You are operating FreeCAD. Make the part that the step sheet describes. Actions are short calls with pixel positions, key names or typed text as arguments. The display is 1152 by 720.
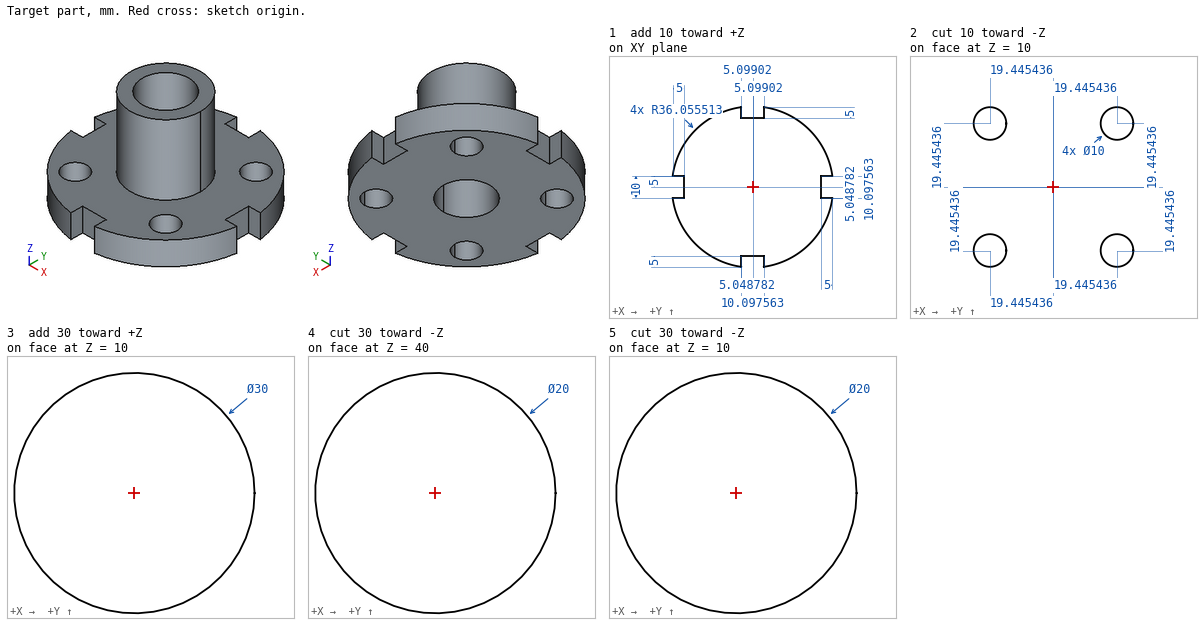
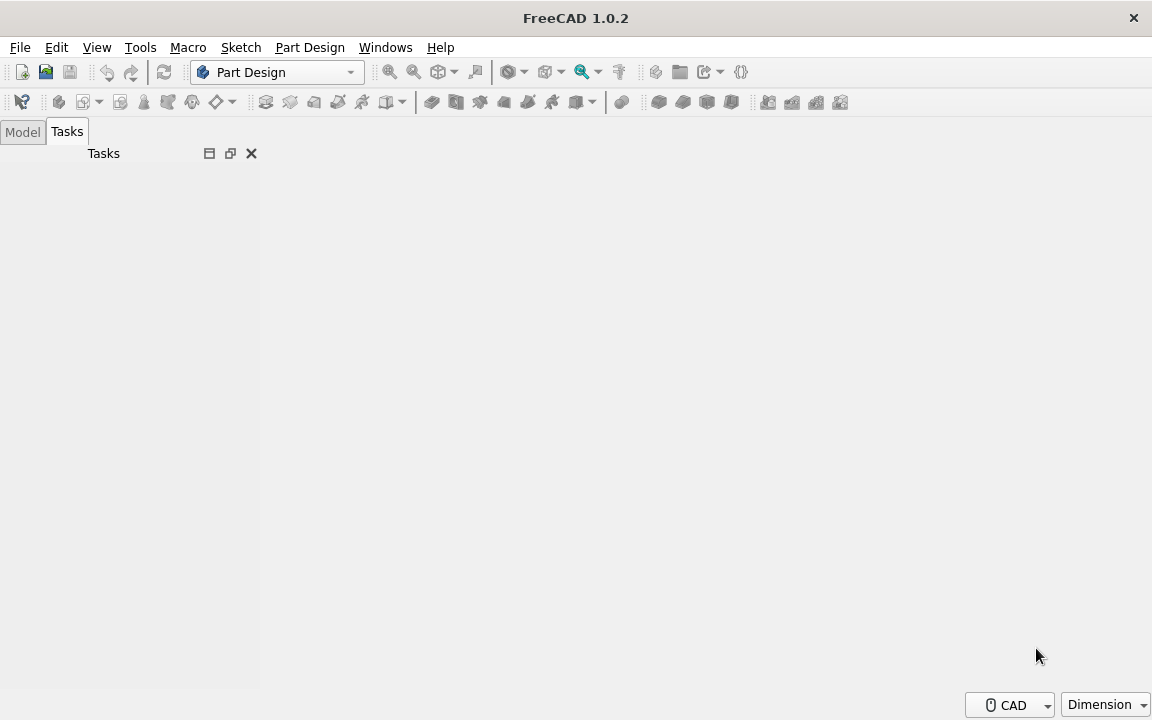
click(22, 72)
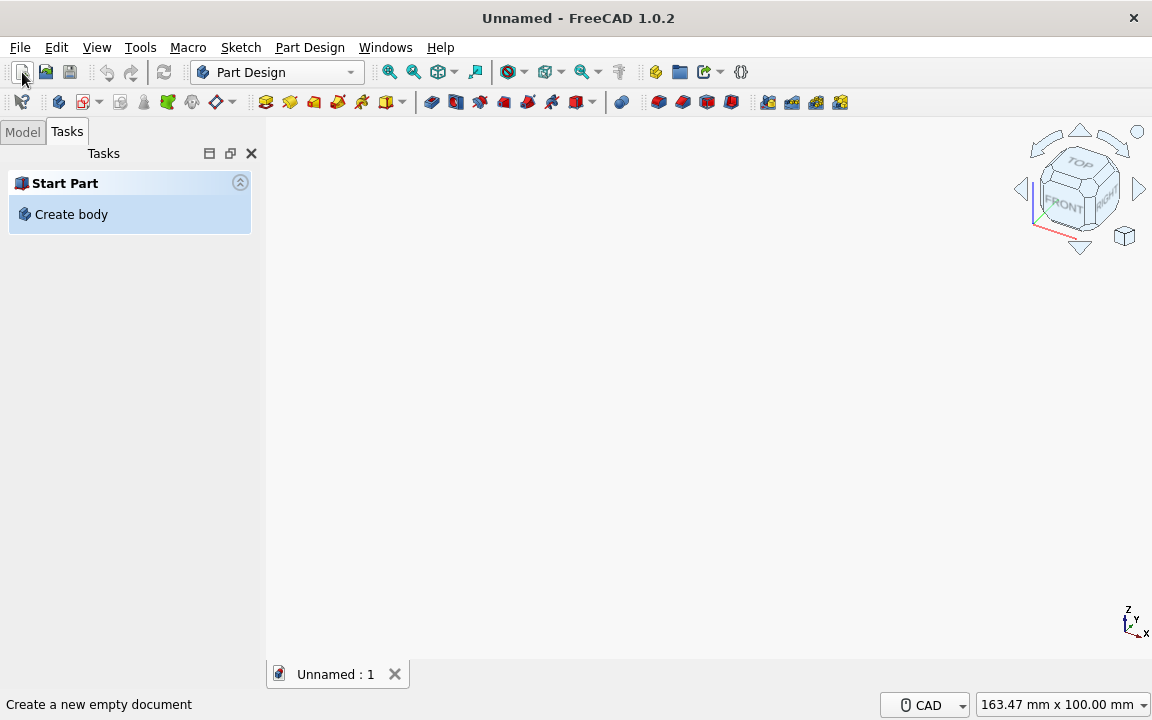
click(84, 102)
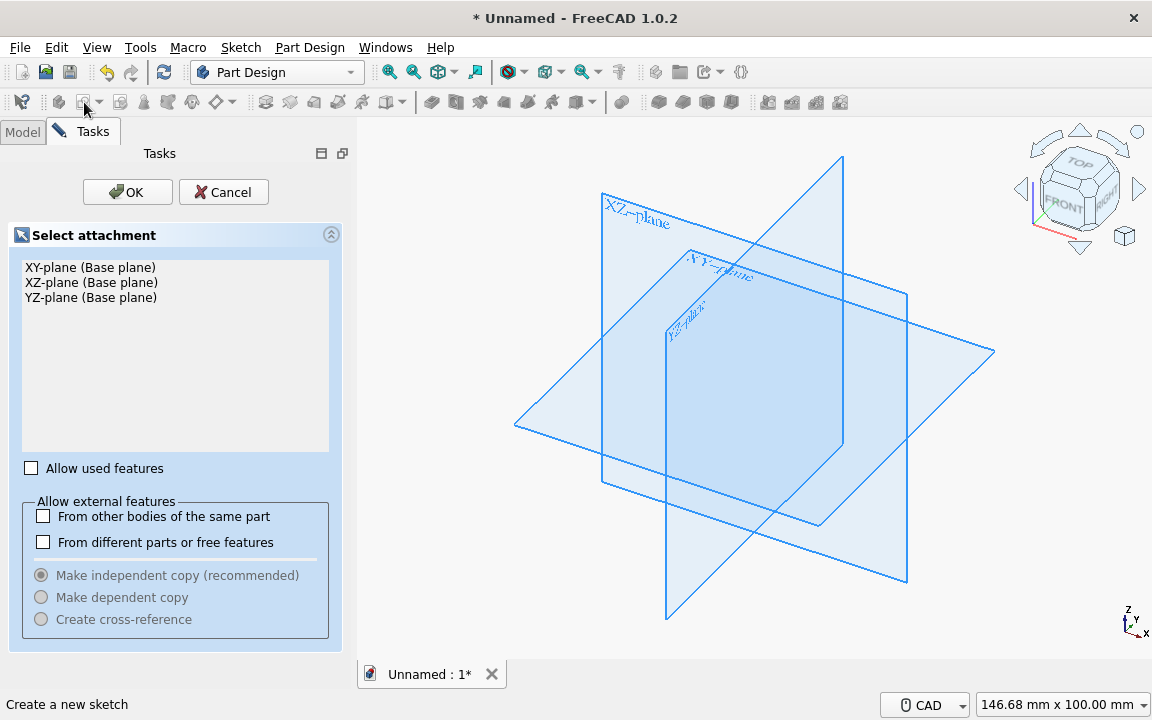
click(82, 268)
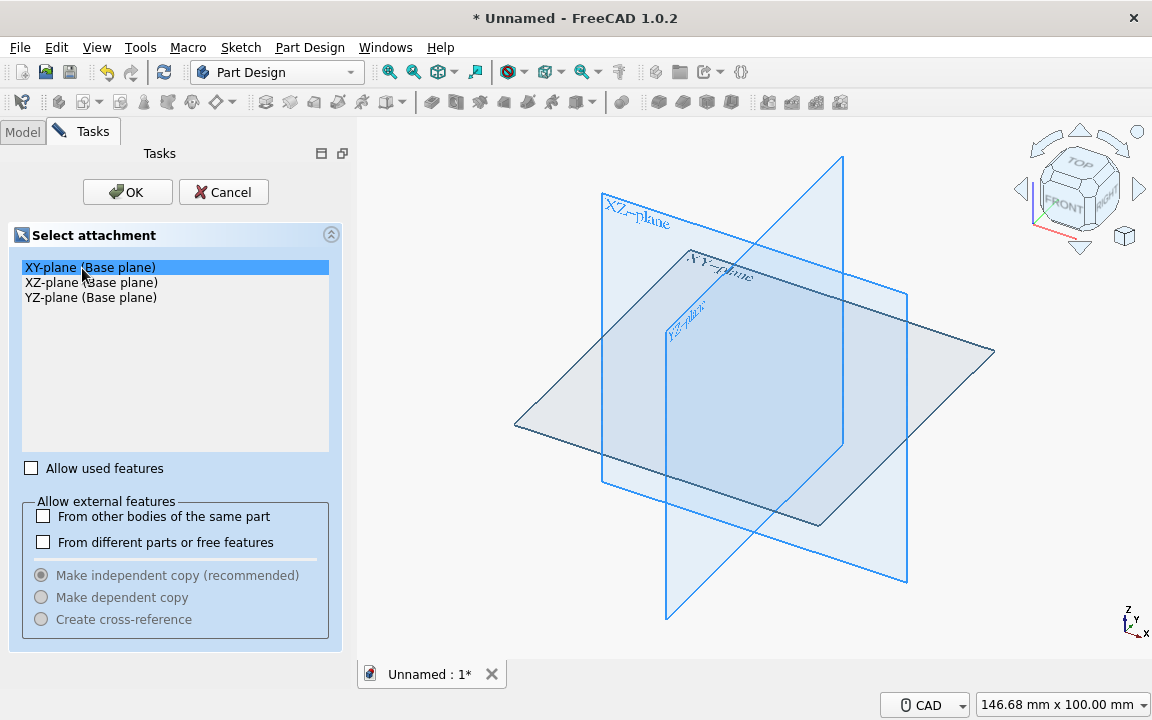
click(128, 192)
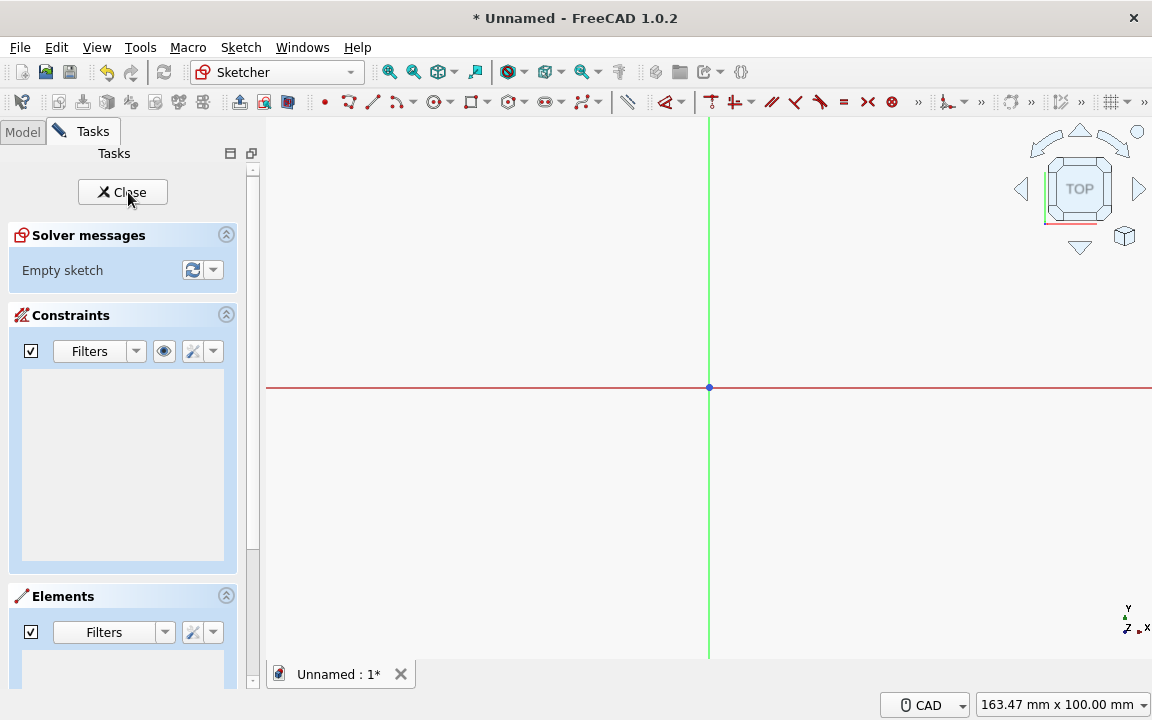
key(g)
key(m)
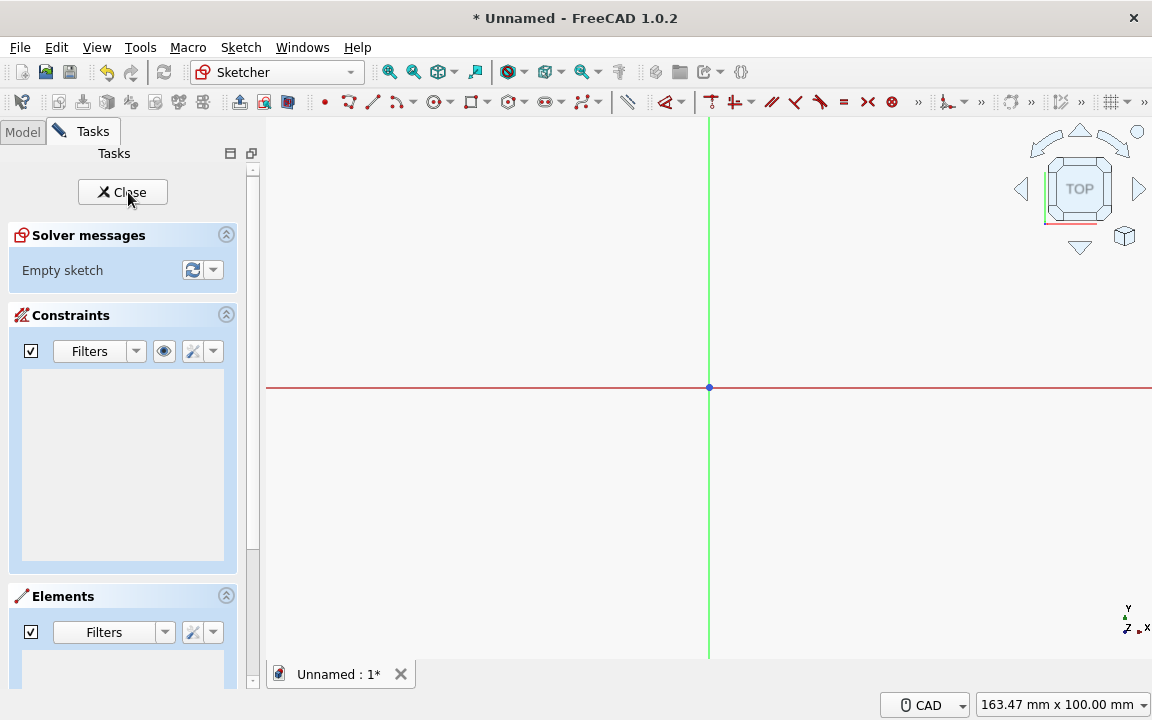
click(737, 195)
click(737, 222)
click(681, 222)
click(681, 195)
right_click(681, 195)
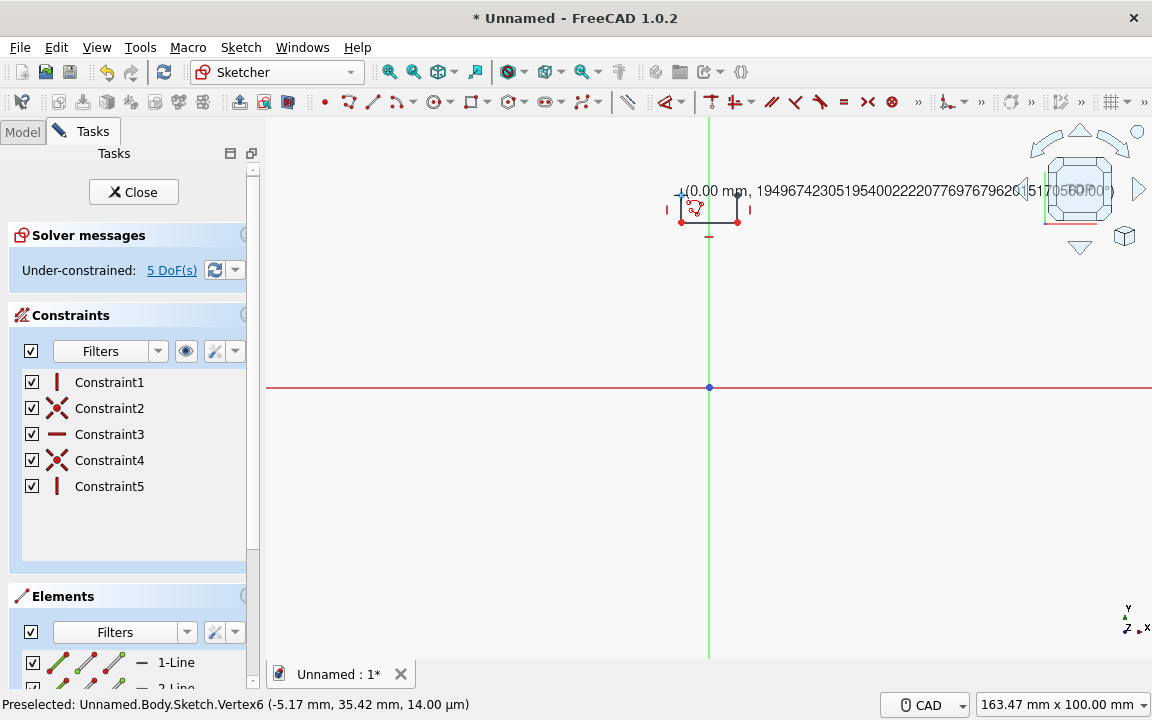
click(515, 361)
click(543, 361)
click(543, 415)
click(515, 415)
right_click(515, 415)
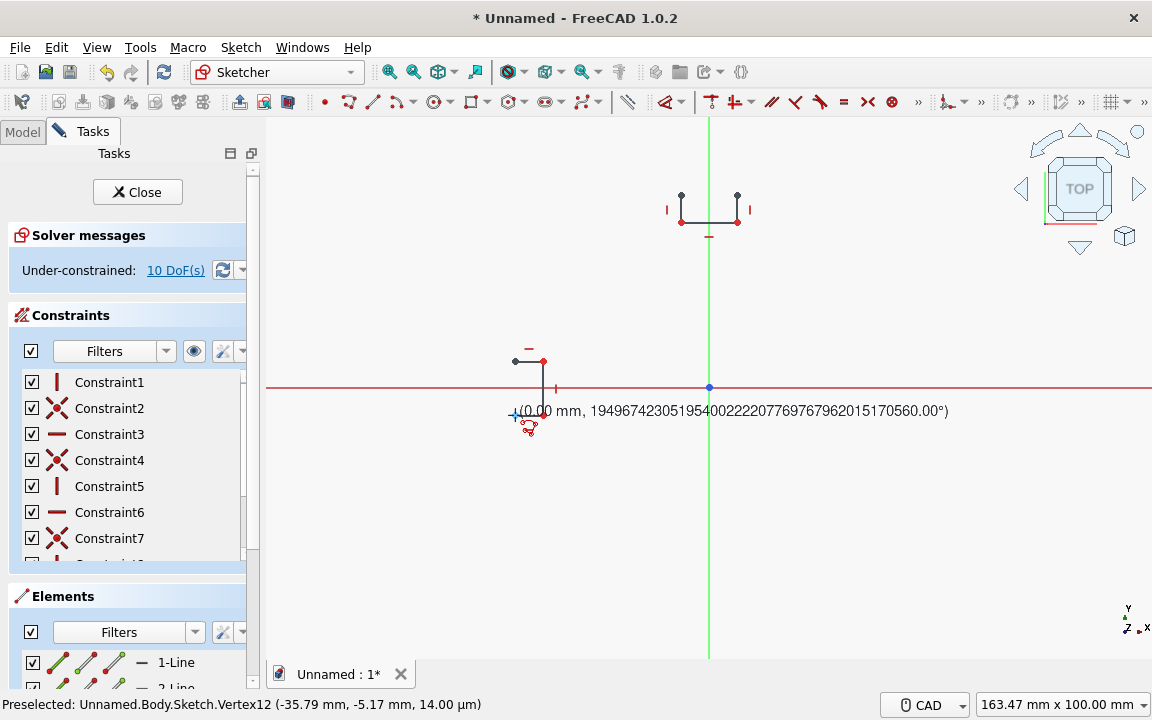
click(682, 581)
click(682, 554)
click(736, 554)
click(736, 581)
right_click(736, 581)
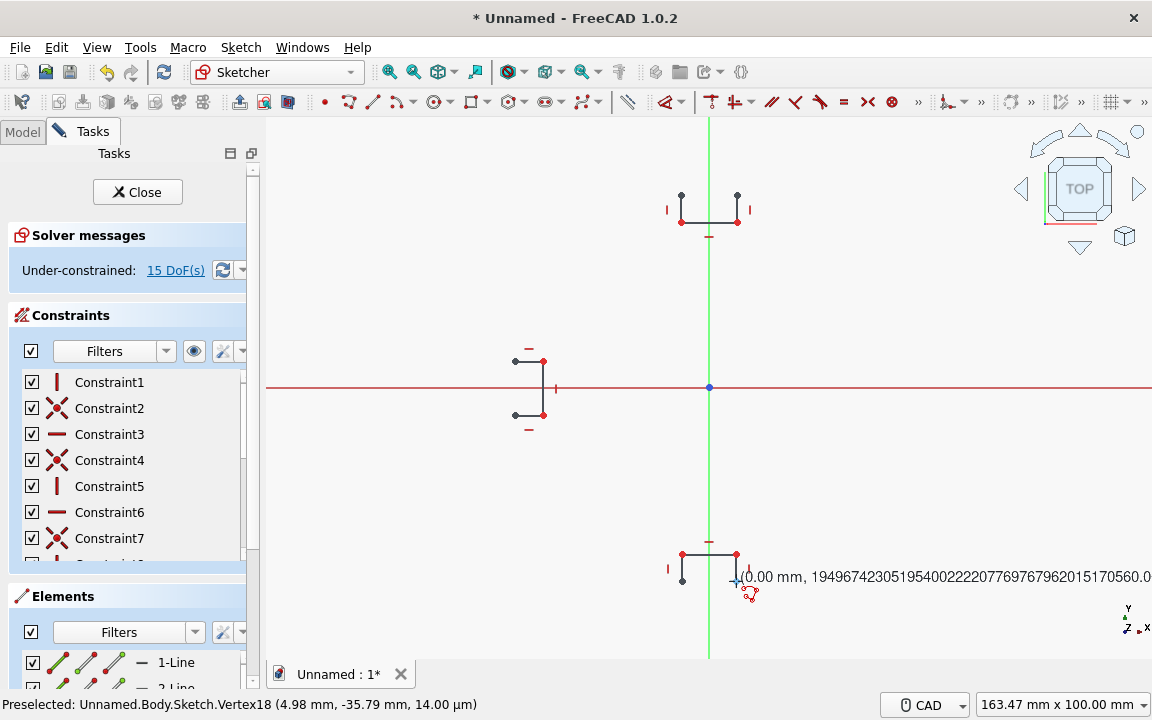
click(902, 415)
click(875, 415)
click(875, 361)
click(902, 361)
right_click(902, 361)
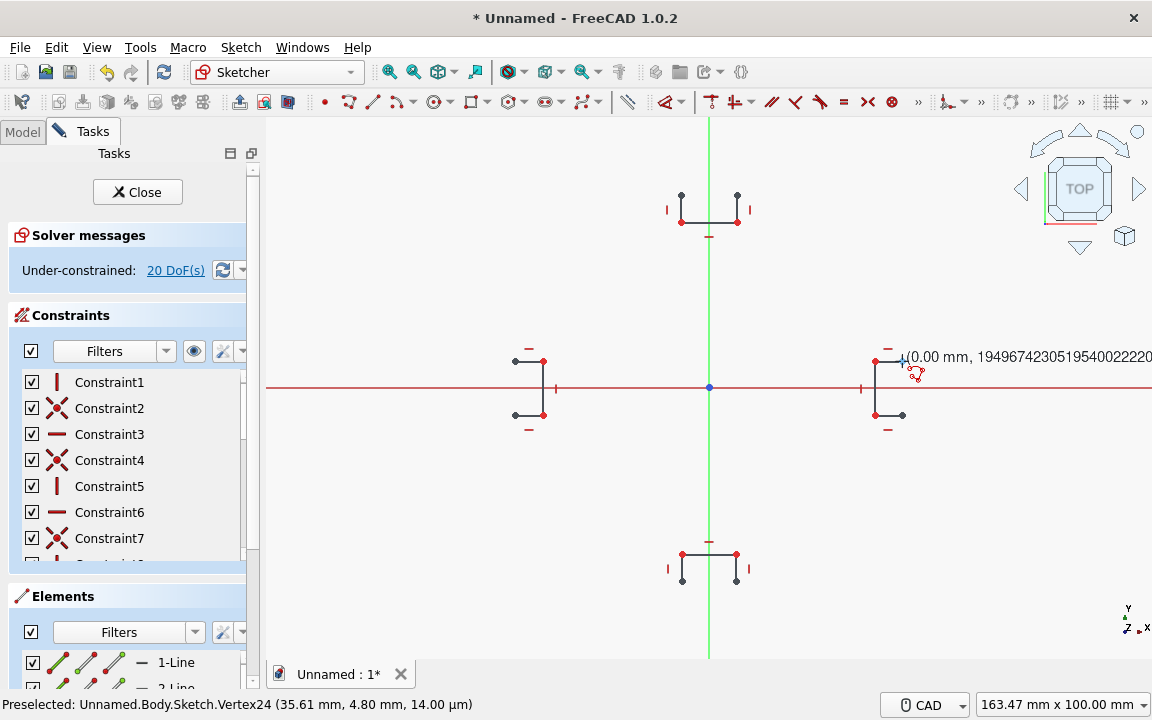
key(g)
key(3)
key(a)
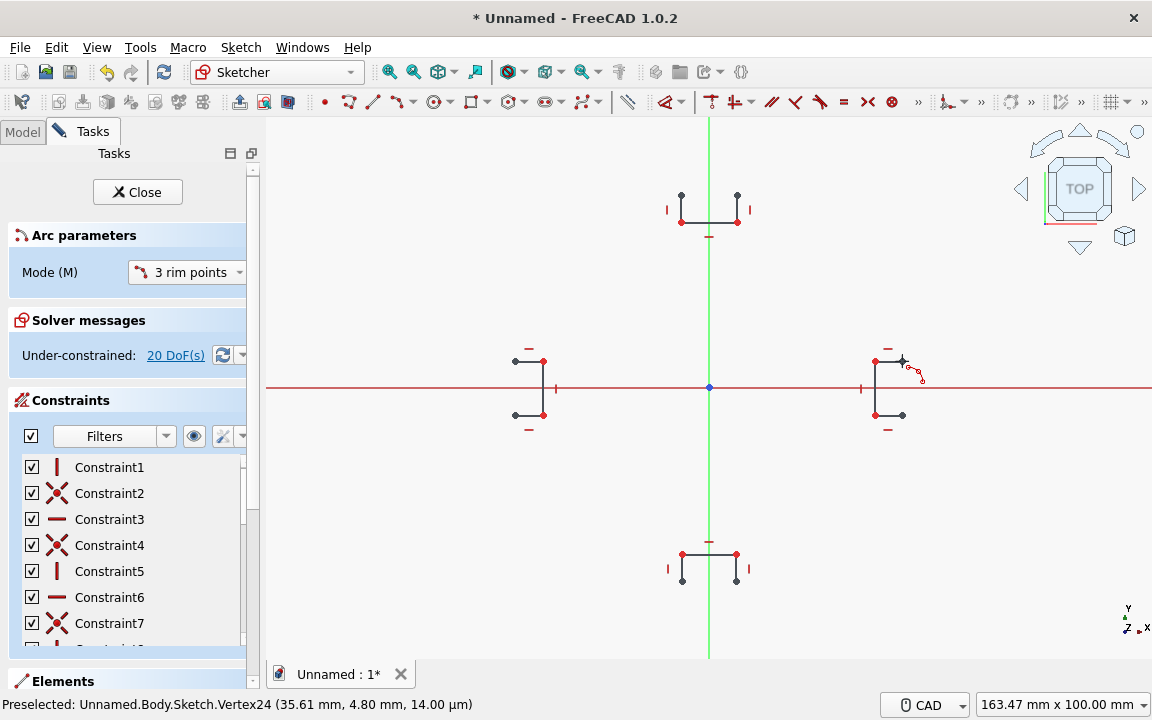
click(681, 196)
click(515, 362)
click(571, 250)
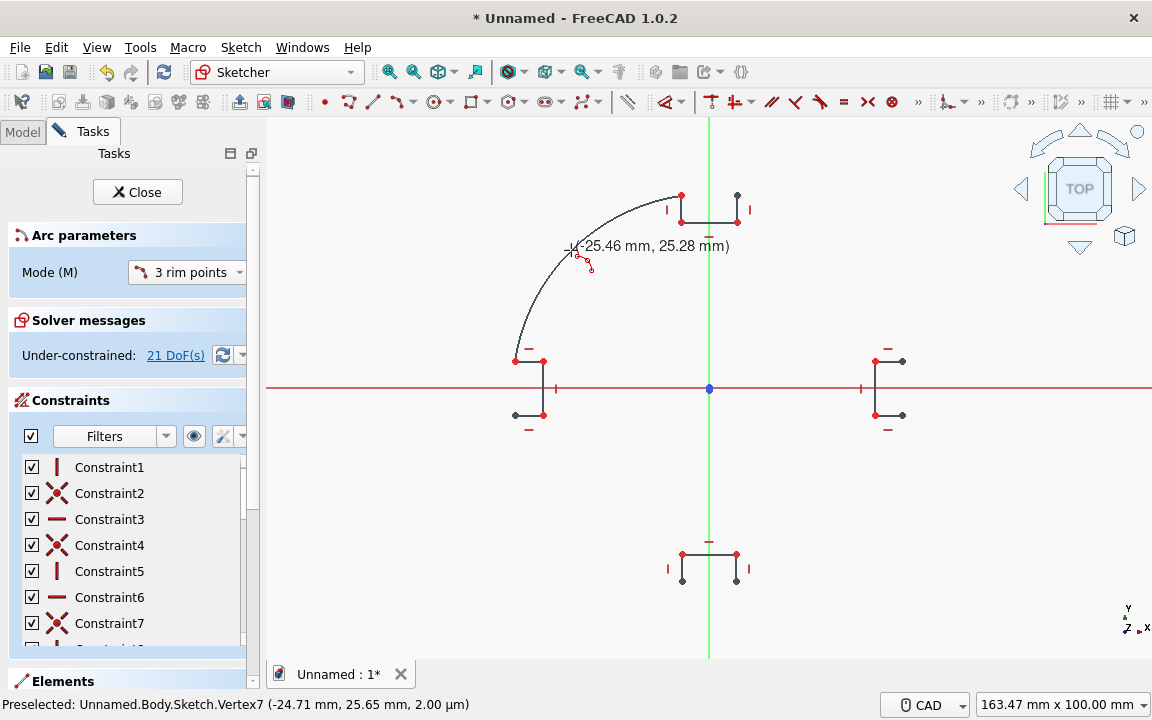
click(515, 416)
click(682, 582)
click(571, 526)